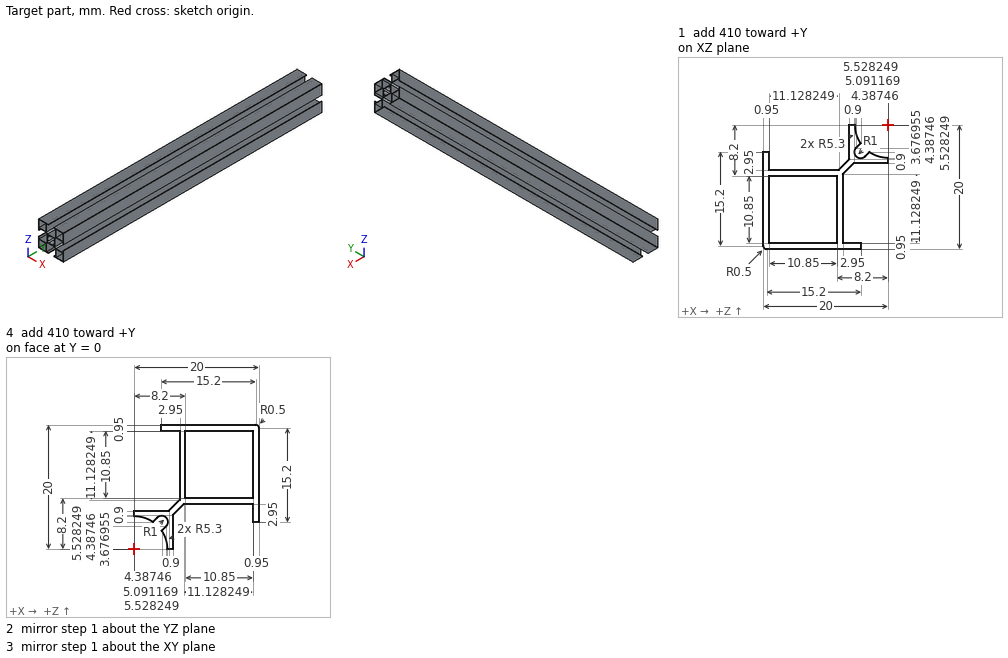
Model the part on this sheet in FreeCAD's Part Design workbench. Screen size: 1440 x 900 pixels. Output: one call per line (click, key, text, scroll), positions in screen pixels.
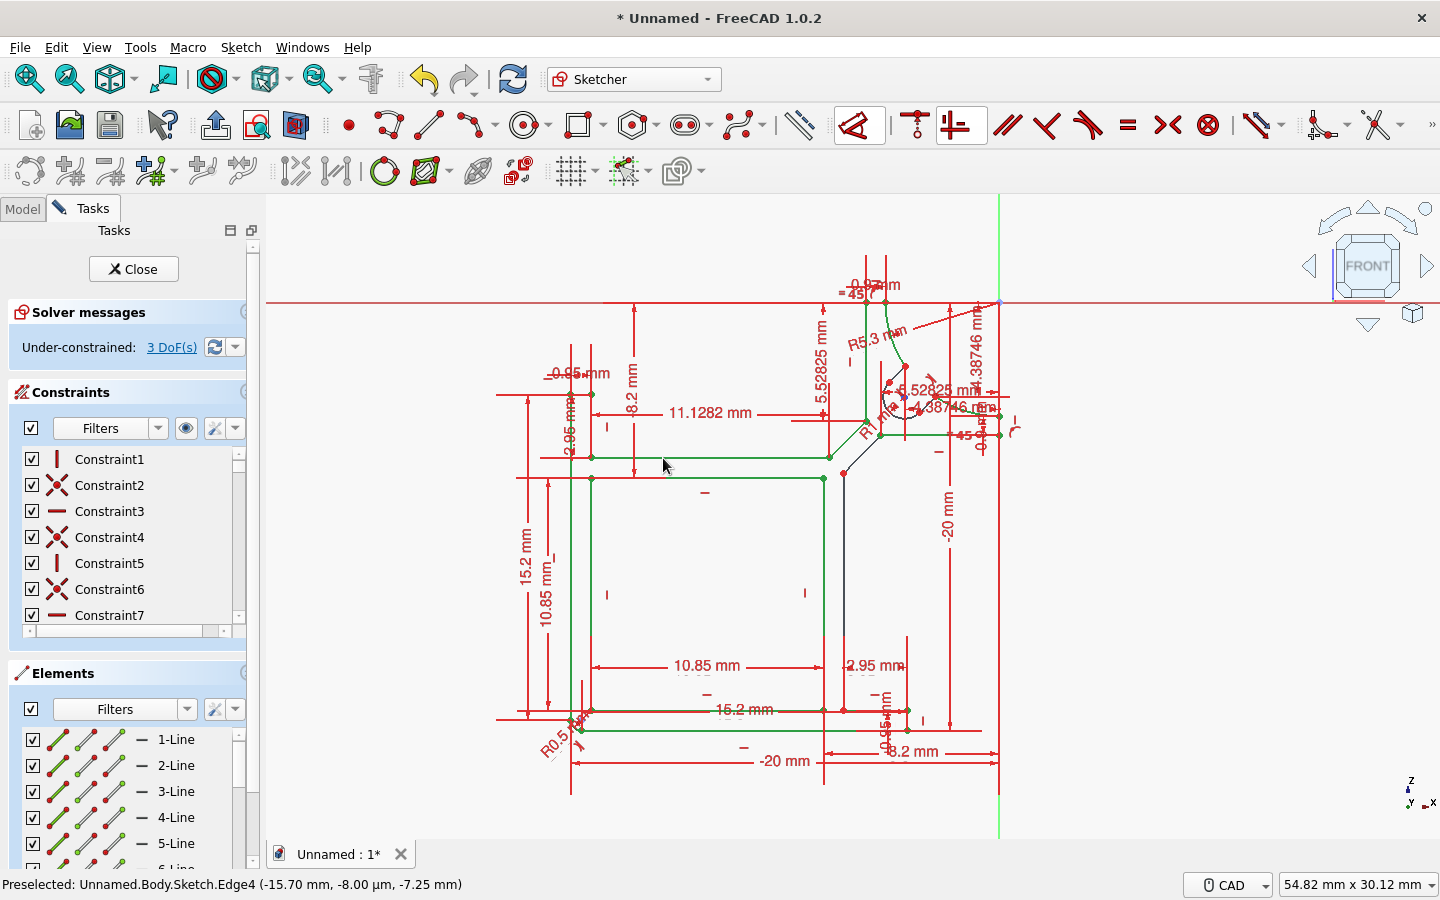
click(844, 544)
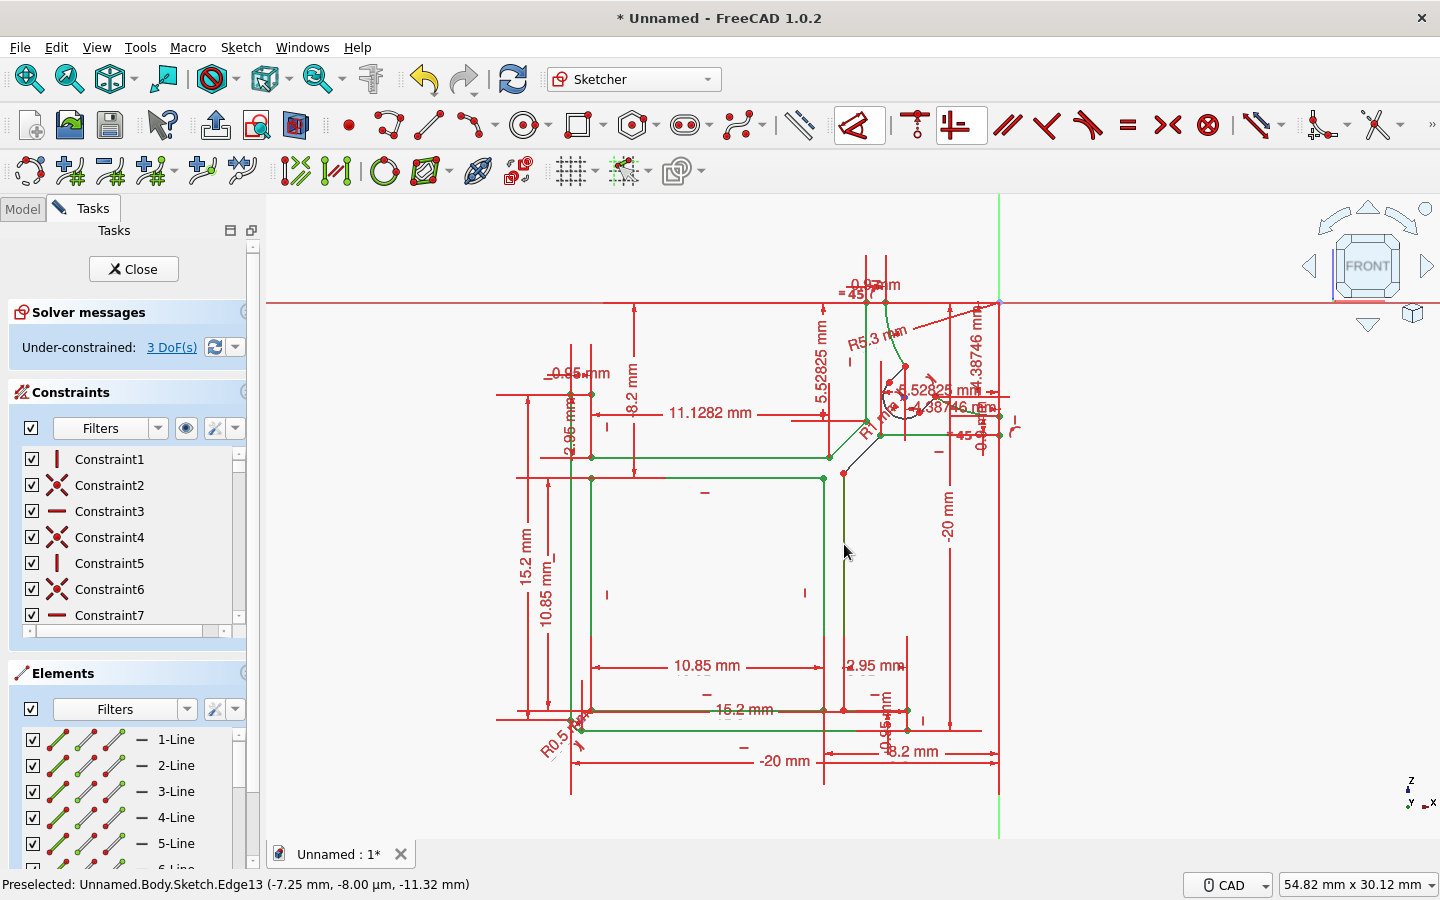
click(880, 126)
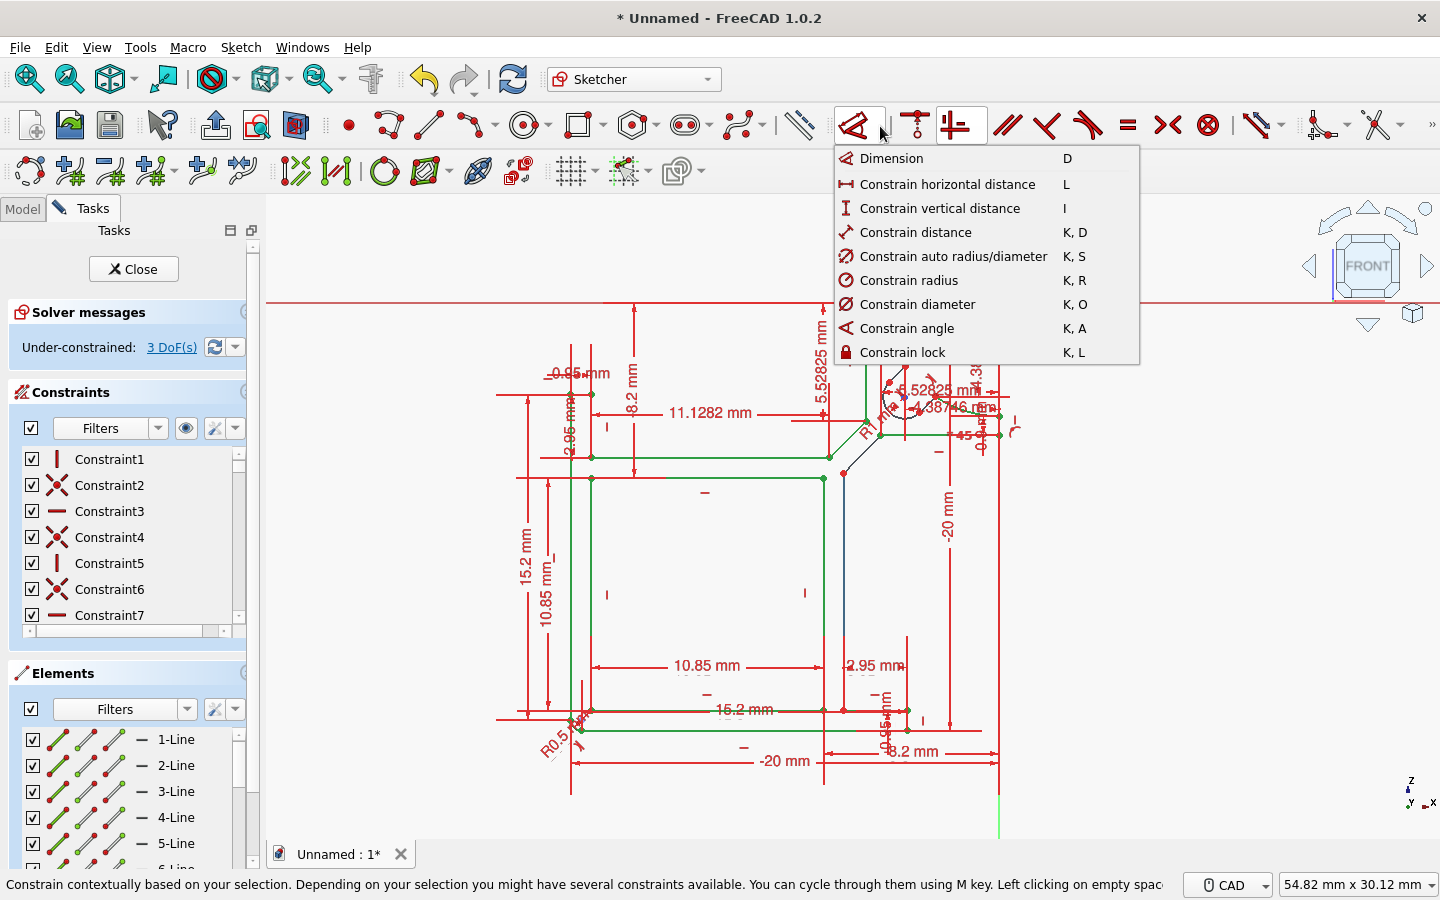
click(987, 208)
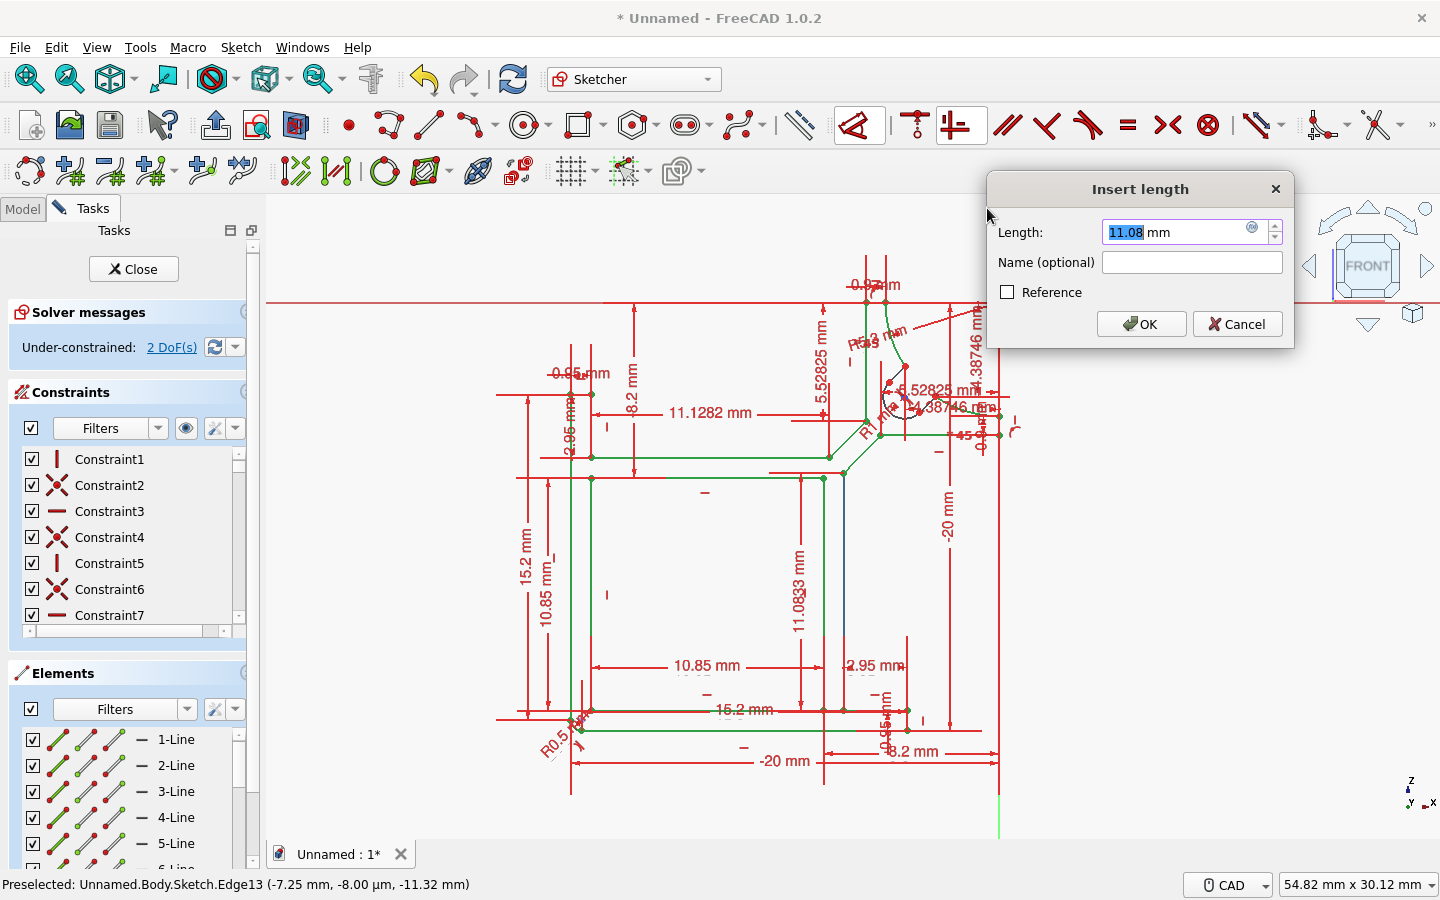
text(11.128249)
key(Return)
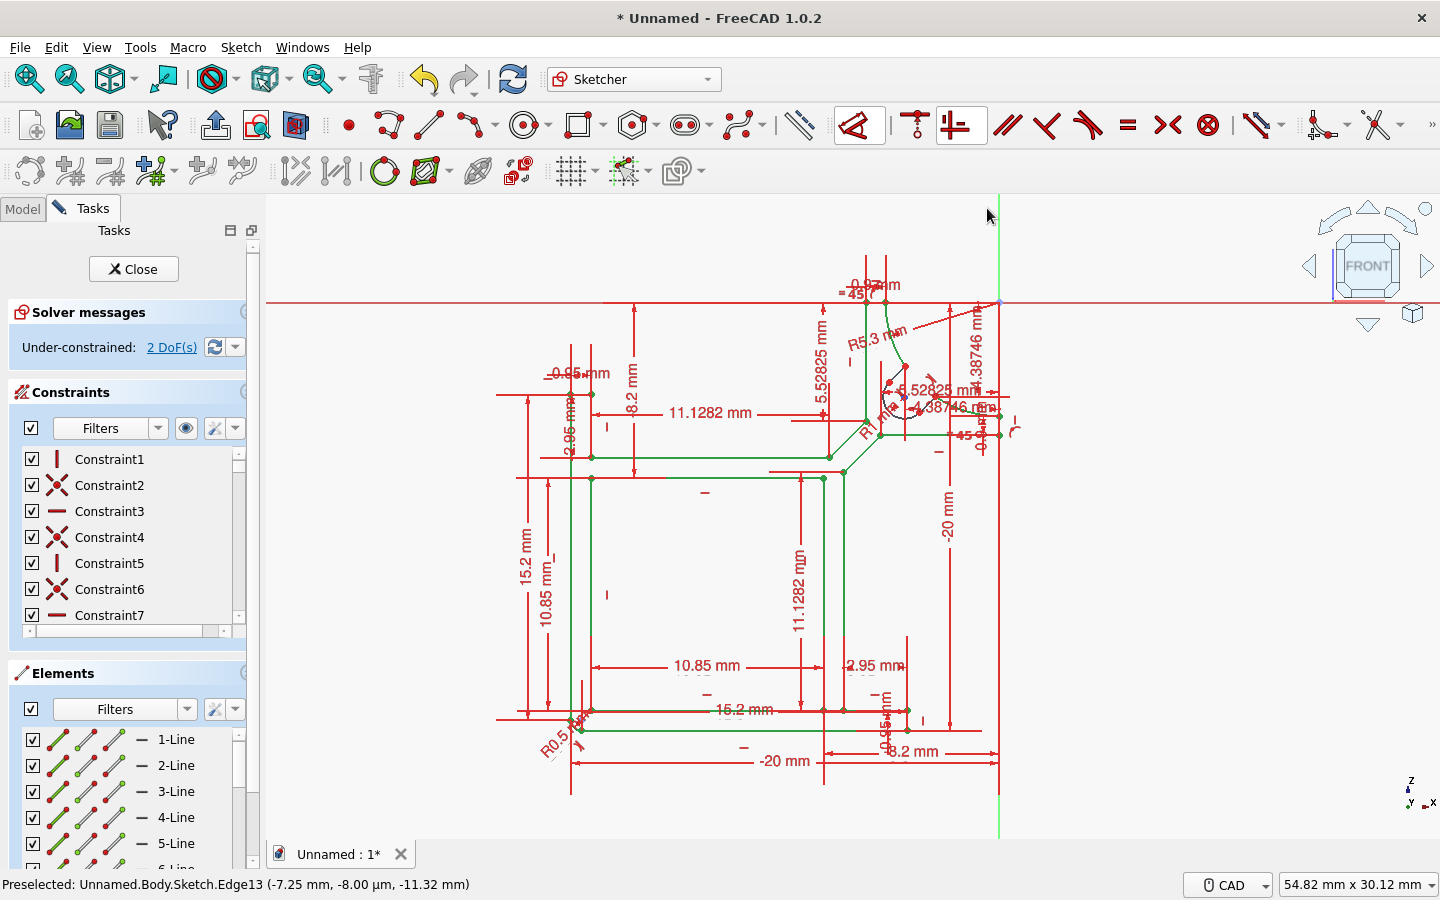
click(889, 382)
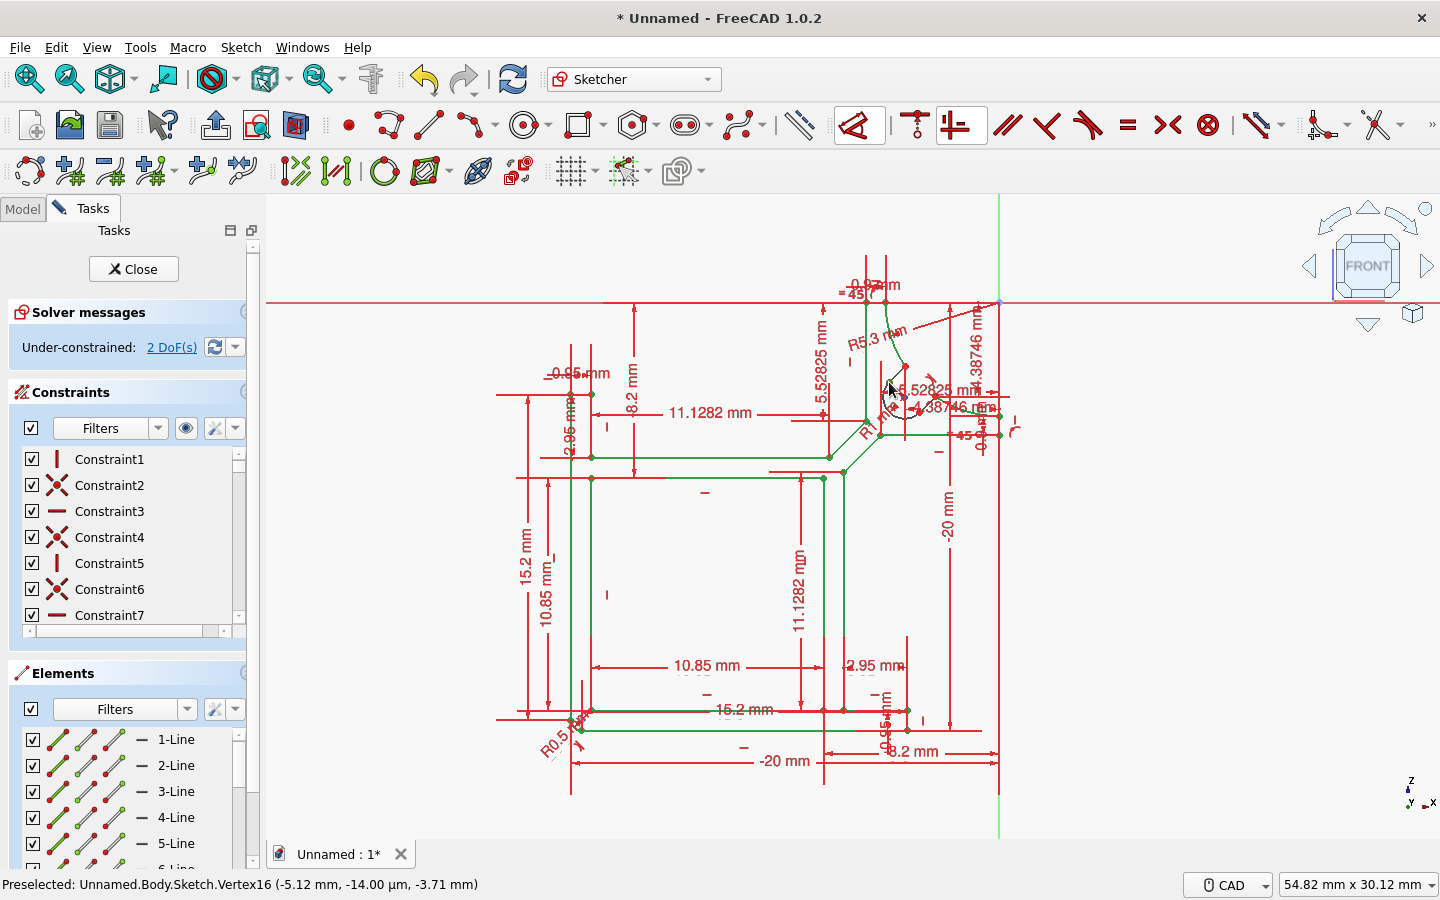
key(l)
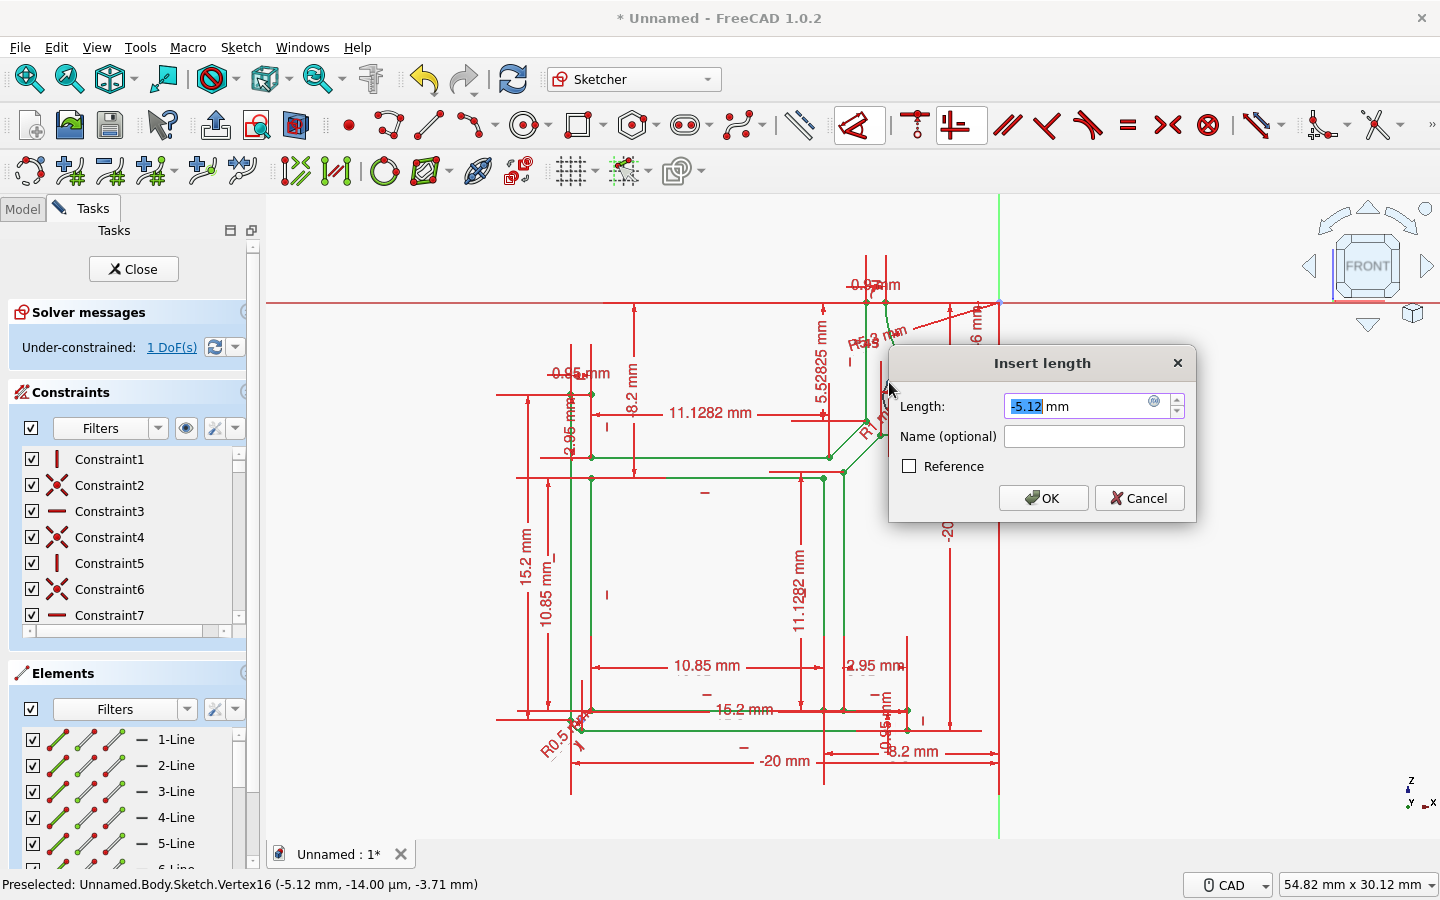
text(-5.091169)
key(Return)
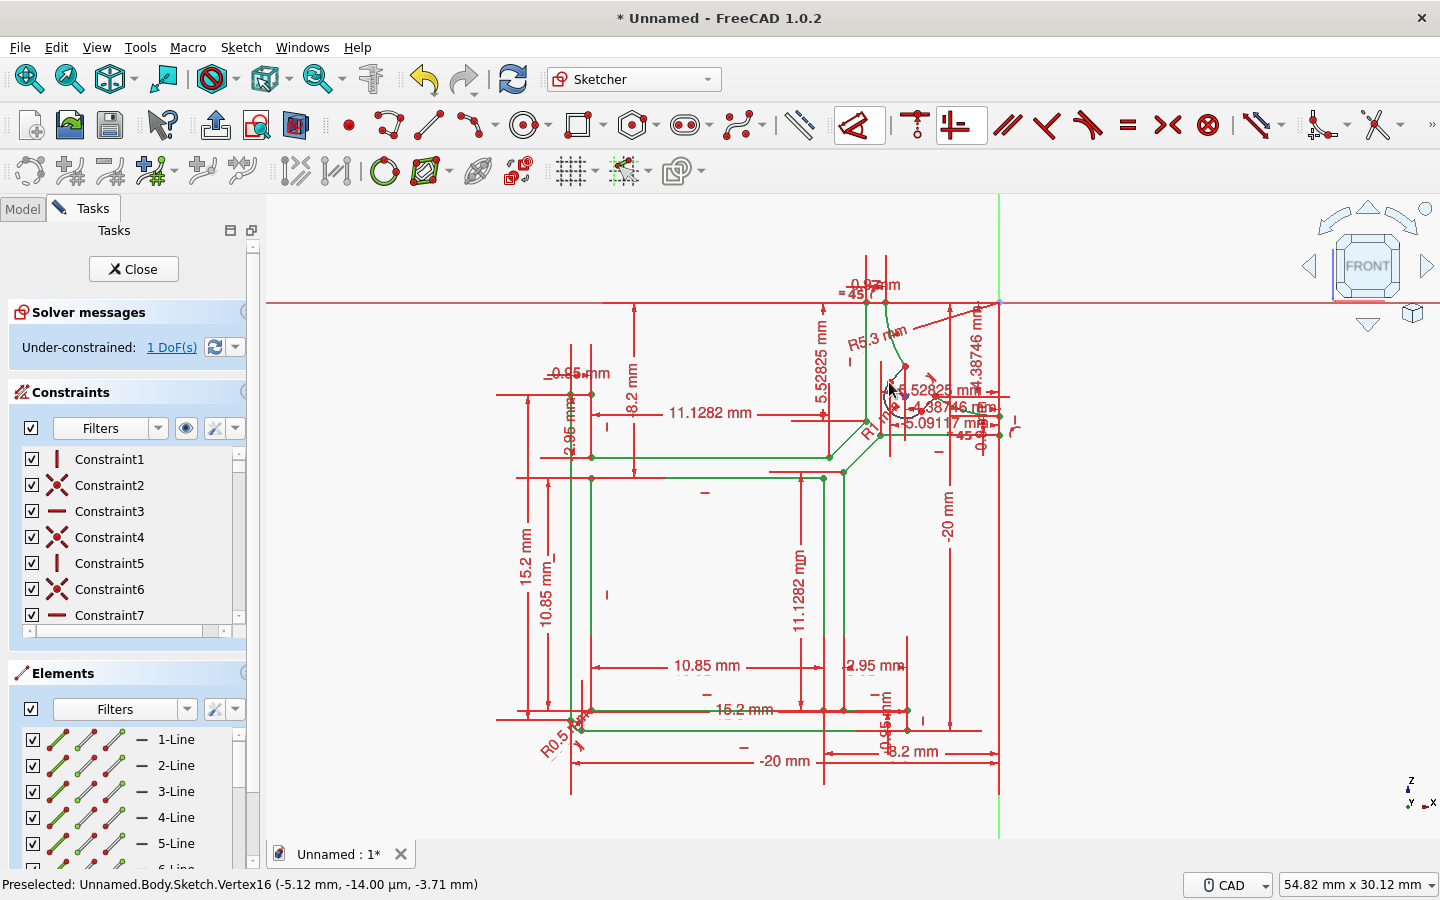
click(890, 382)